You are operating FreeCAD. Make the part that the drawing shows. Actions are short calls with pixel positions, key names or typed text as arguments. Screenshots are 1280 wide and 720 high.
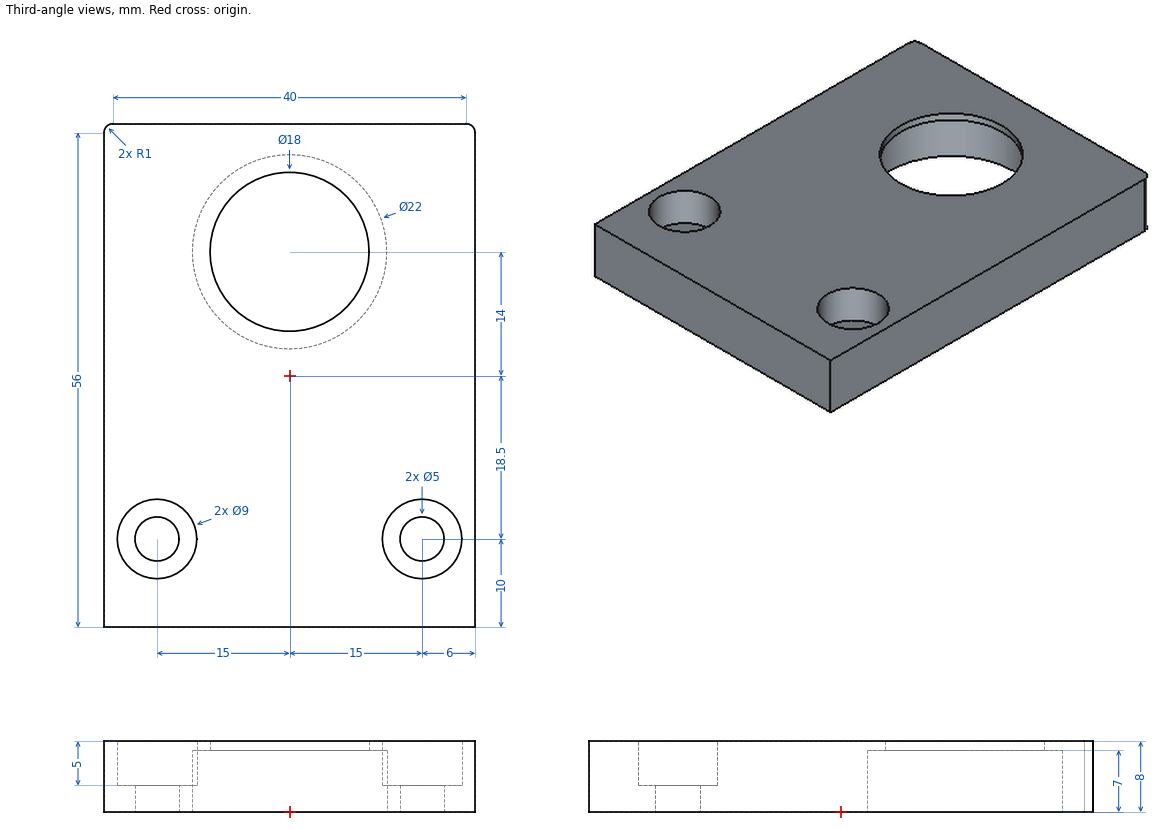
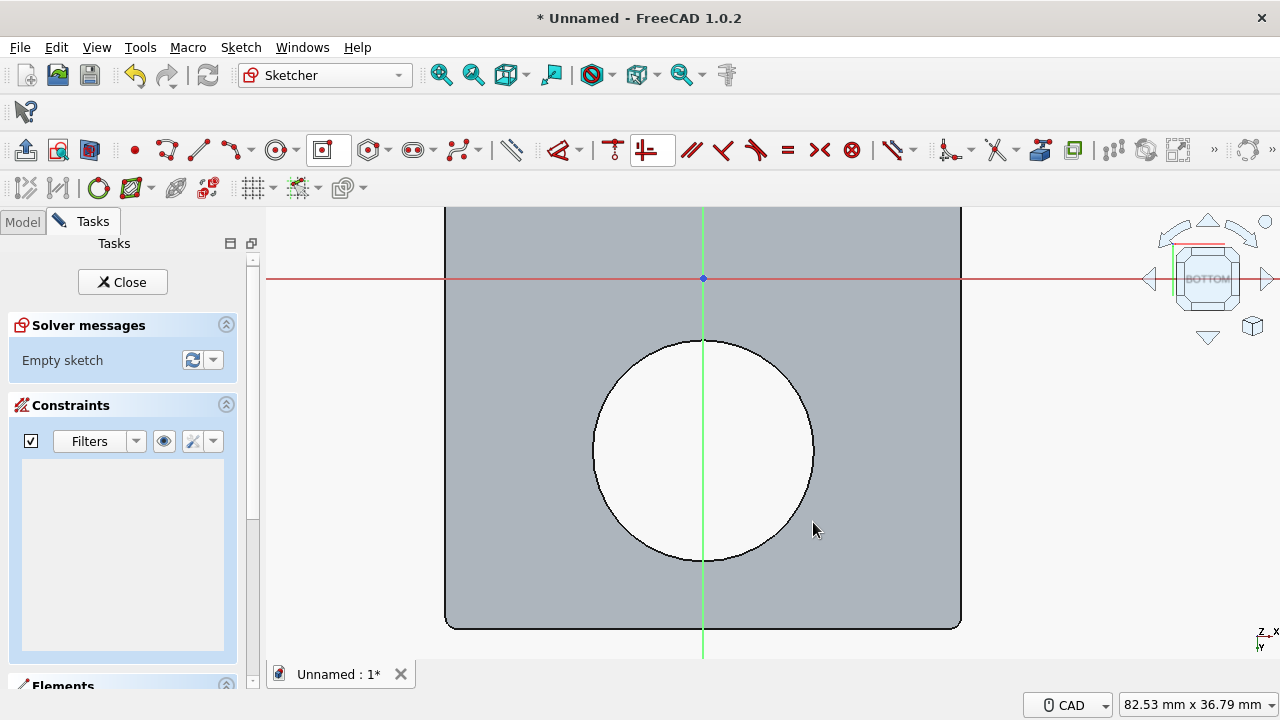
click(276, 150)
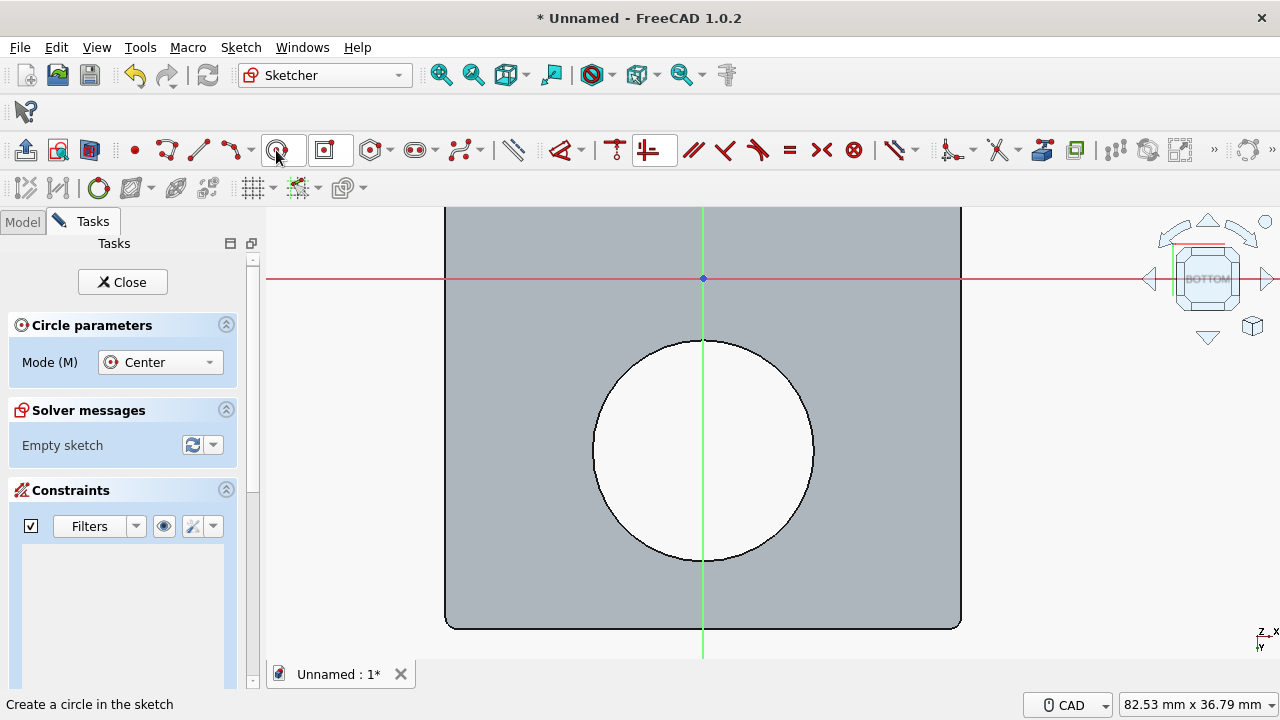
click(703, 451)
click(799, 355)
key(Escape)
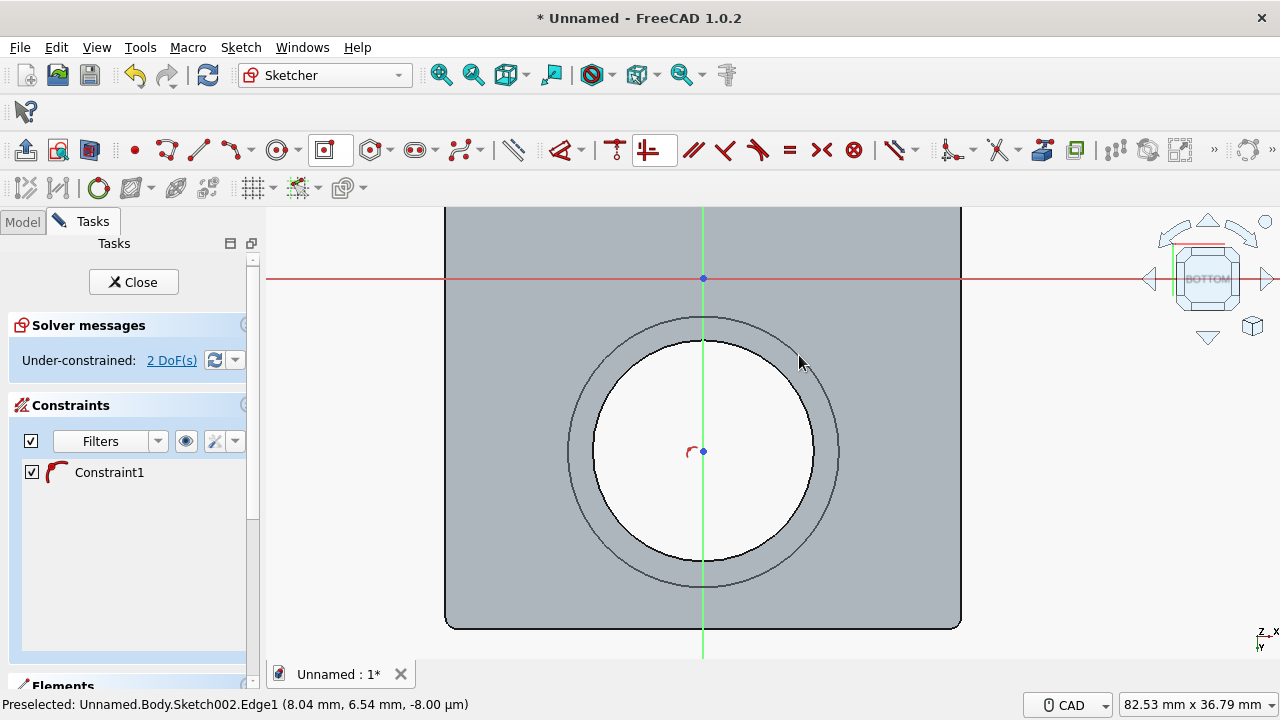
click(560, 150)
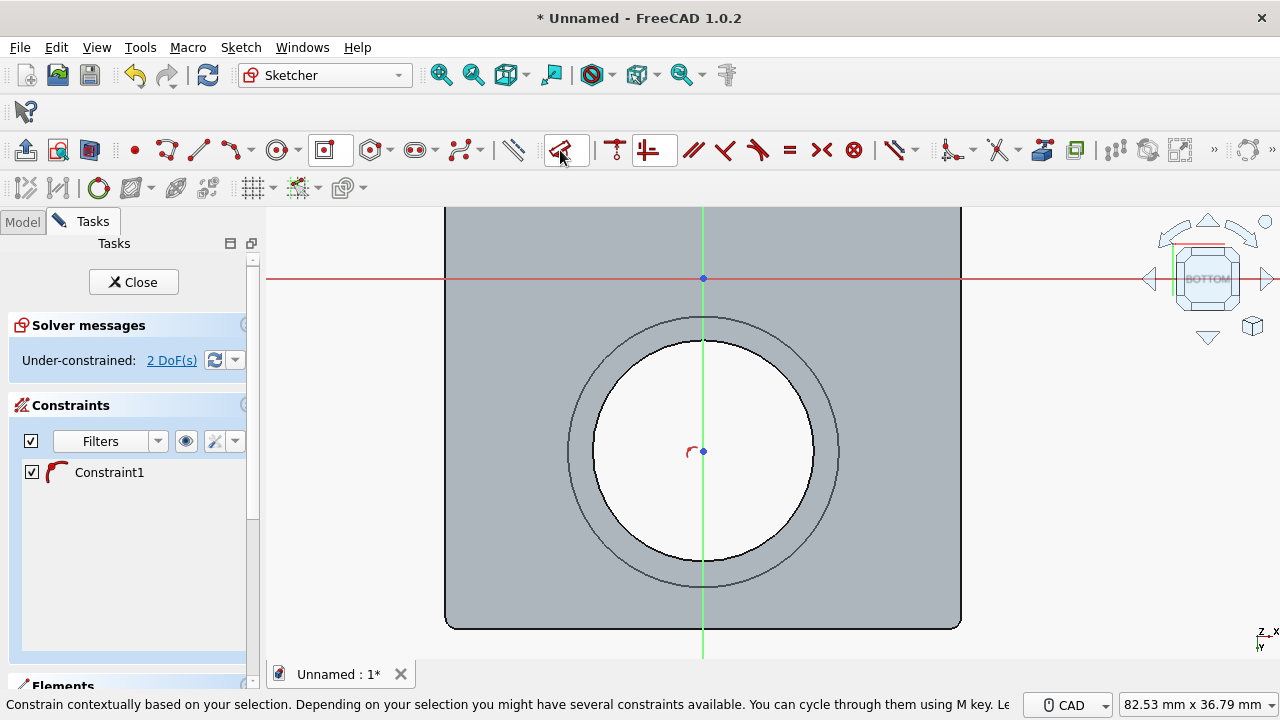
click(799, 356)
click(822, 333)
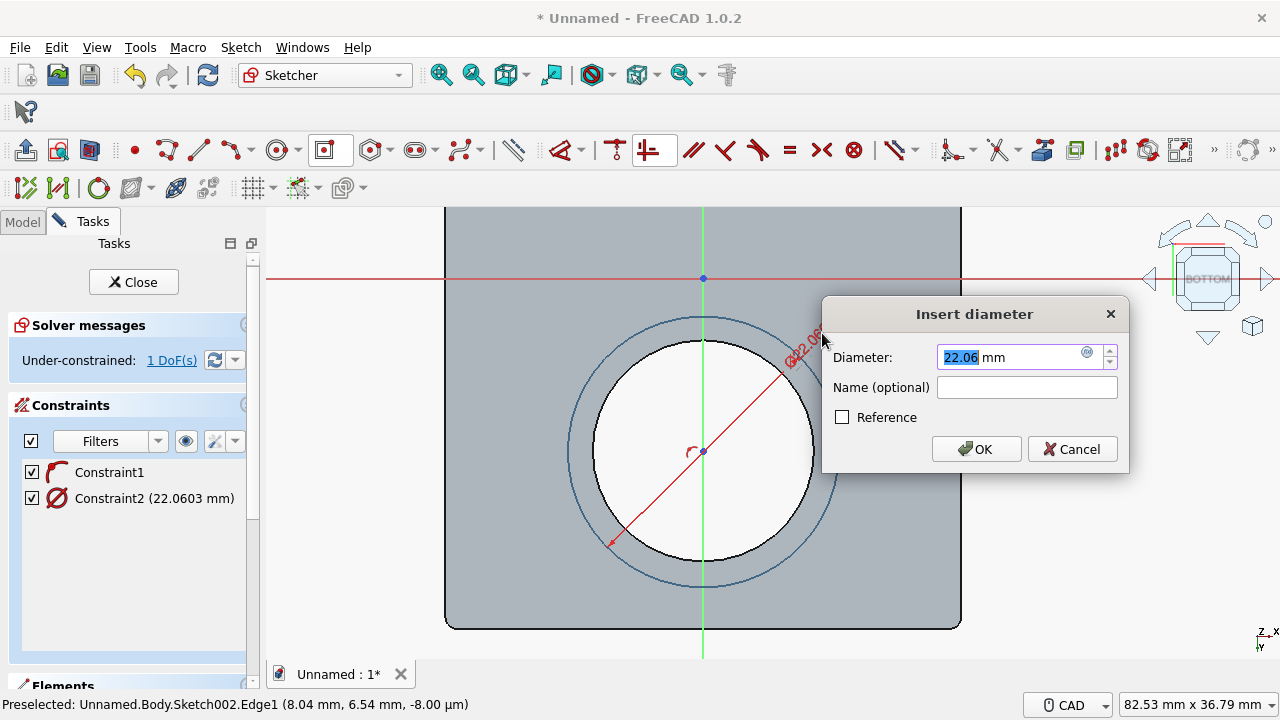
text(22)
key(Return)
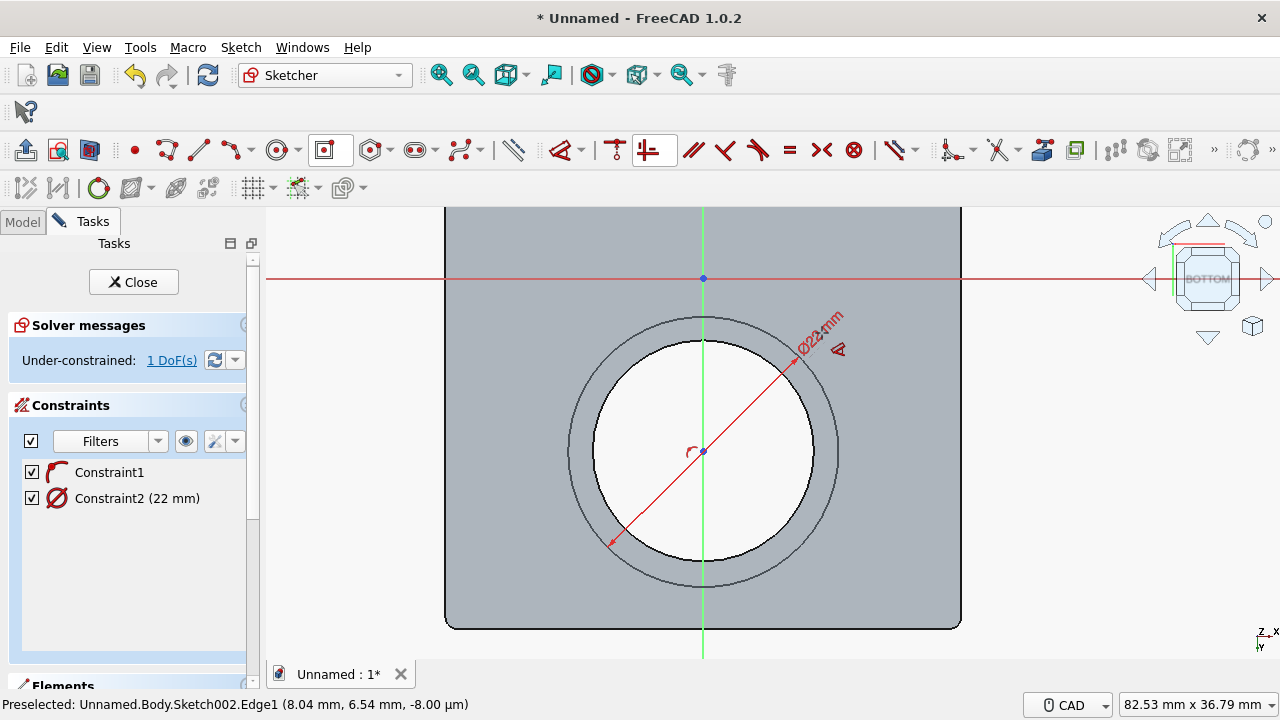
click(703, 452)
click(737, 365)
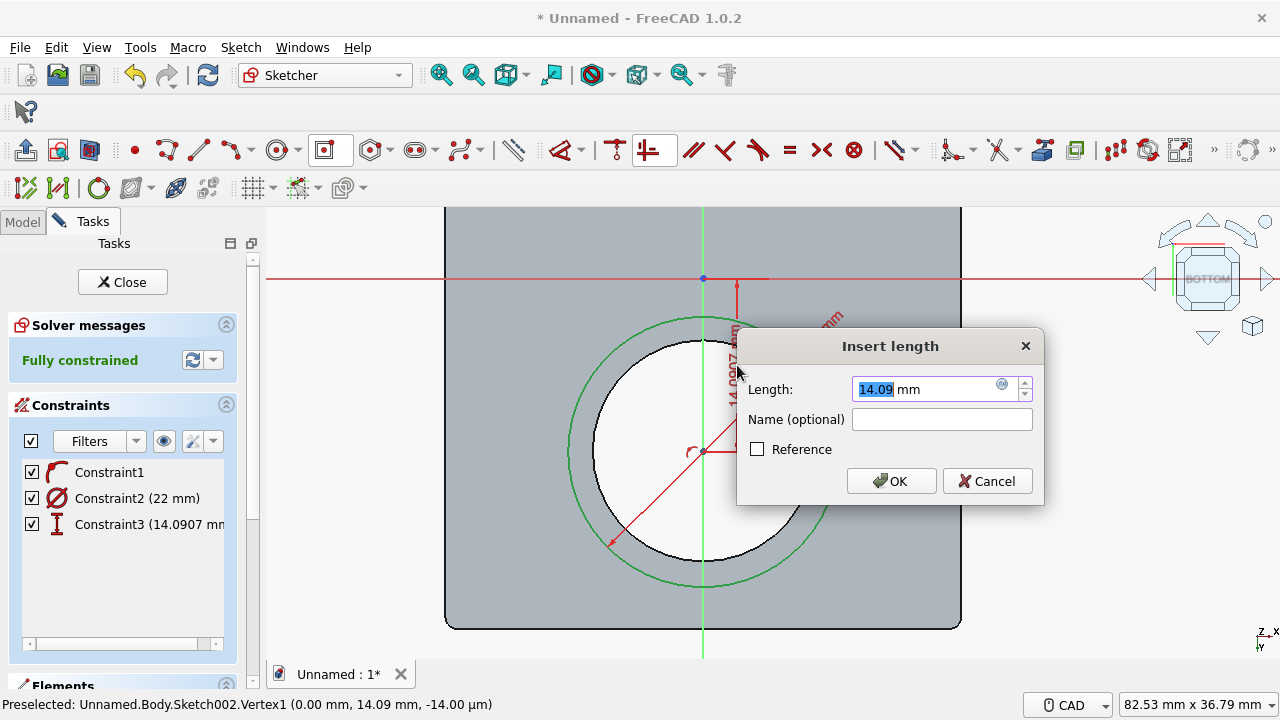
text(14)
key(Return)
key(Escape)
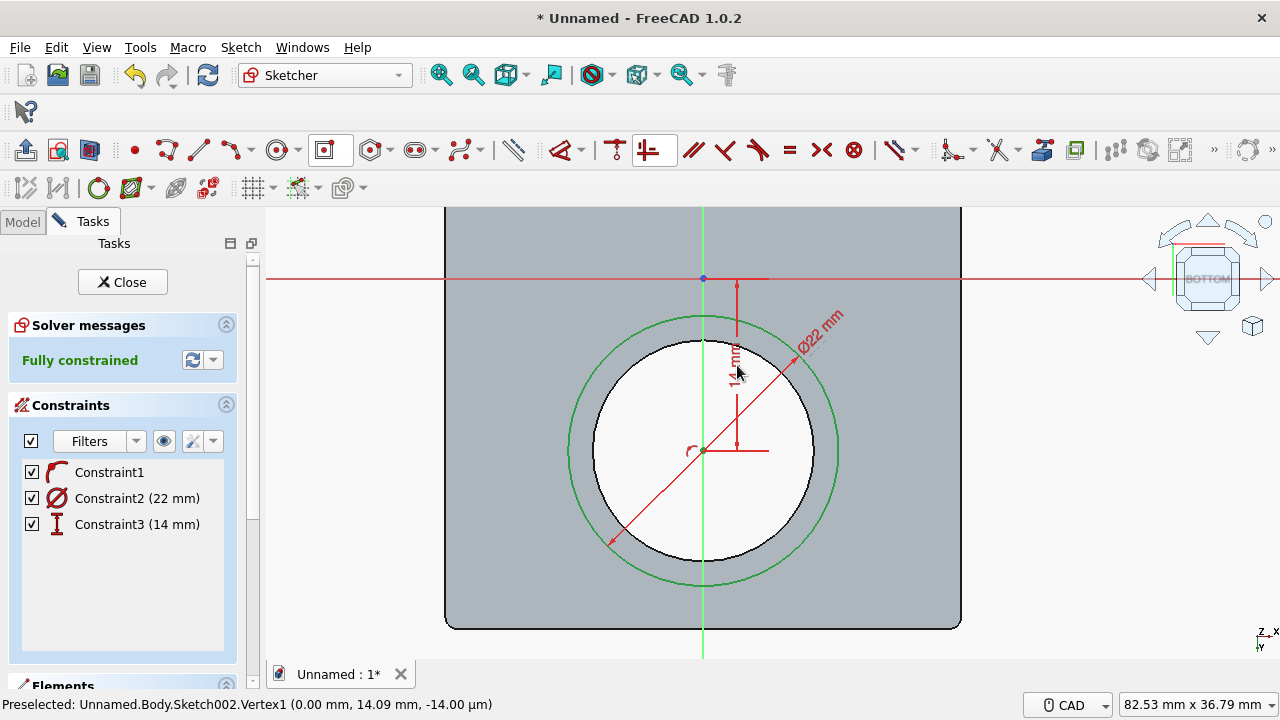
click(123, 282)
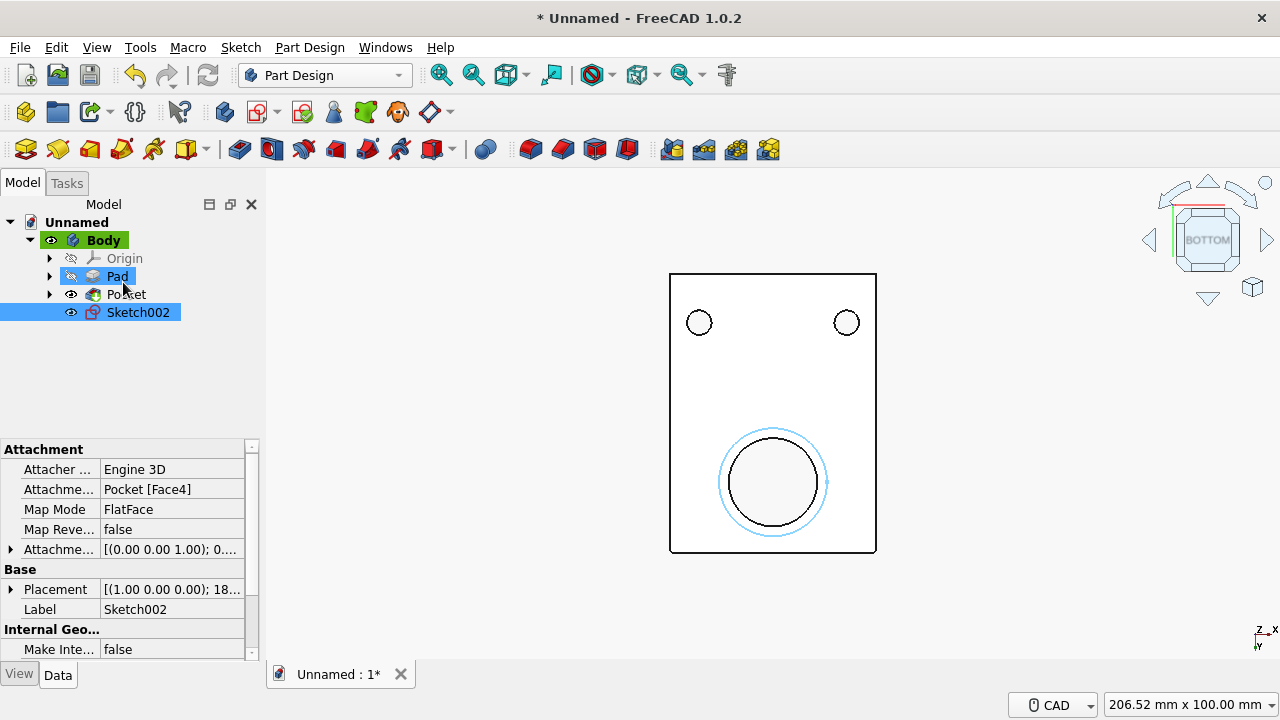
click(240, 150)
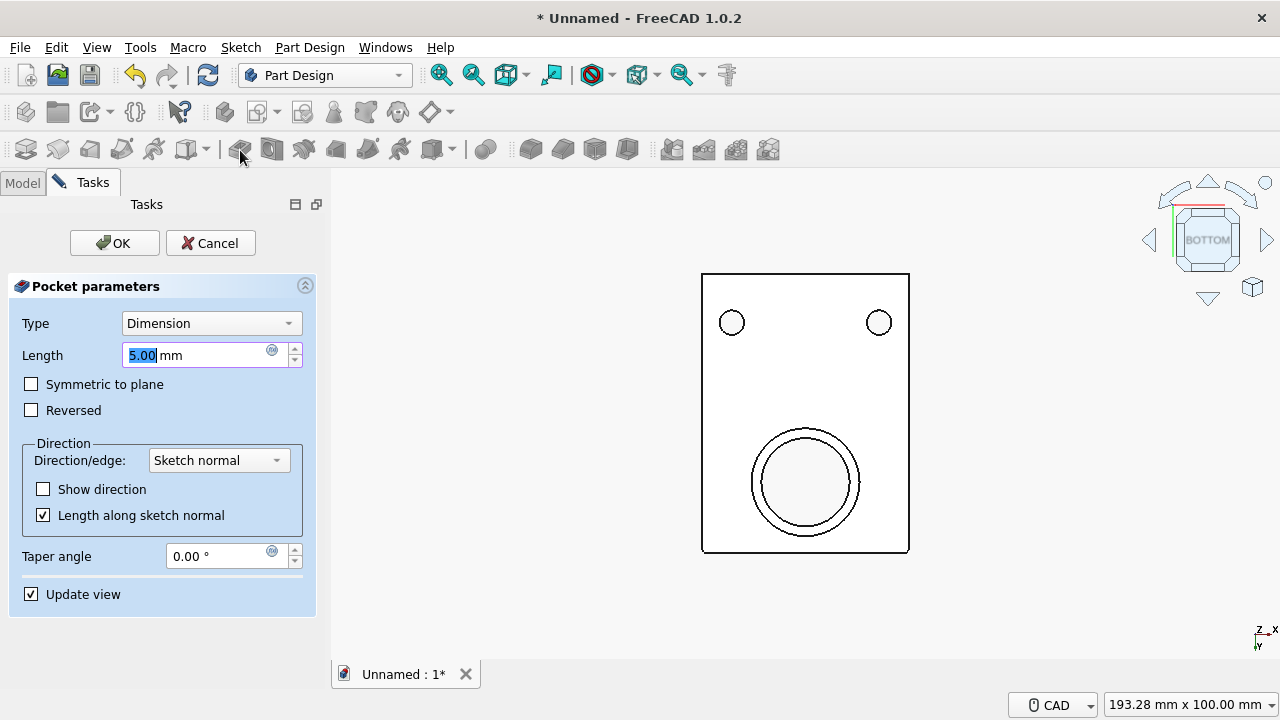
text(7)
key(Tab)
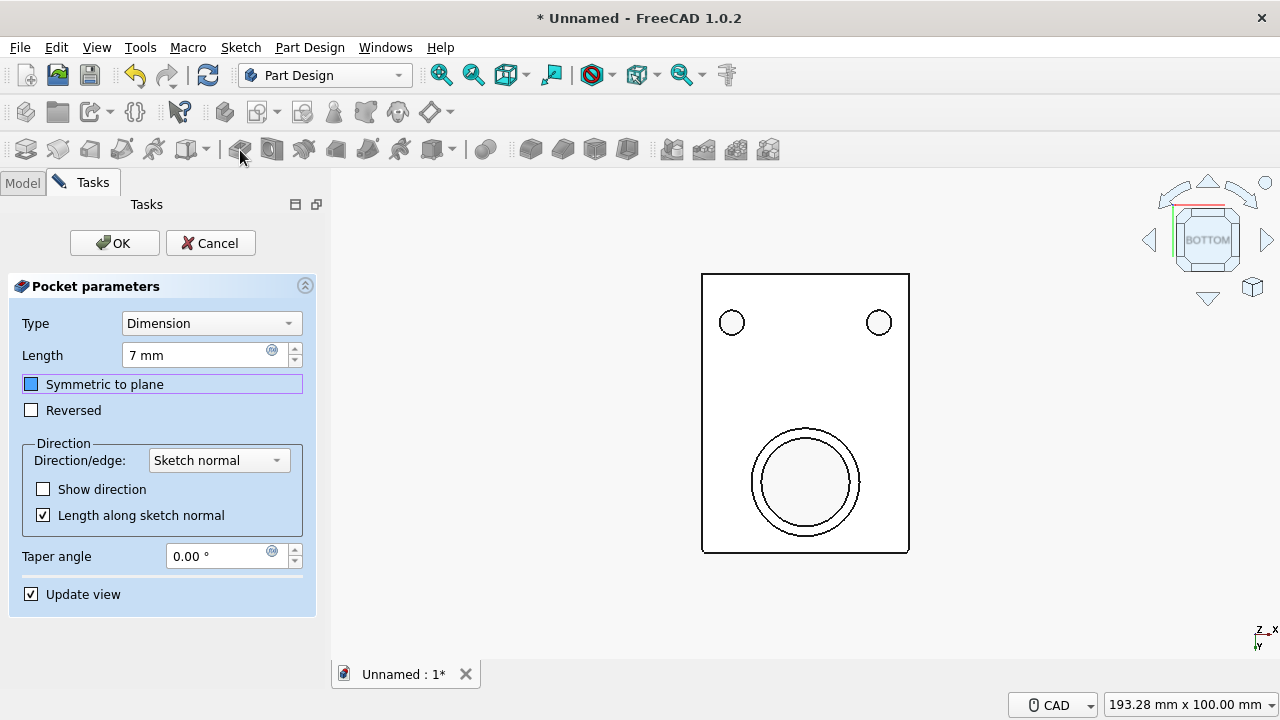
click(115, 243)